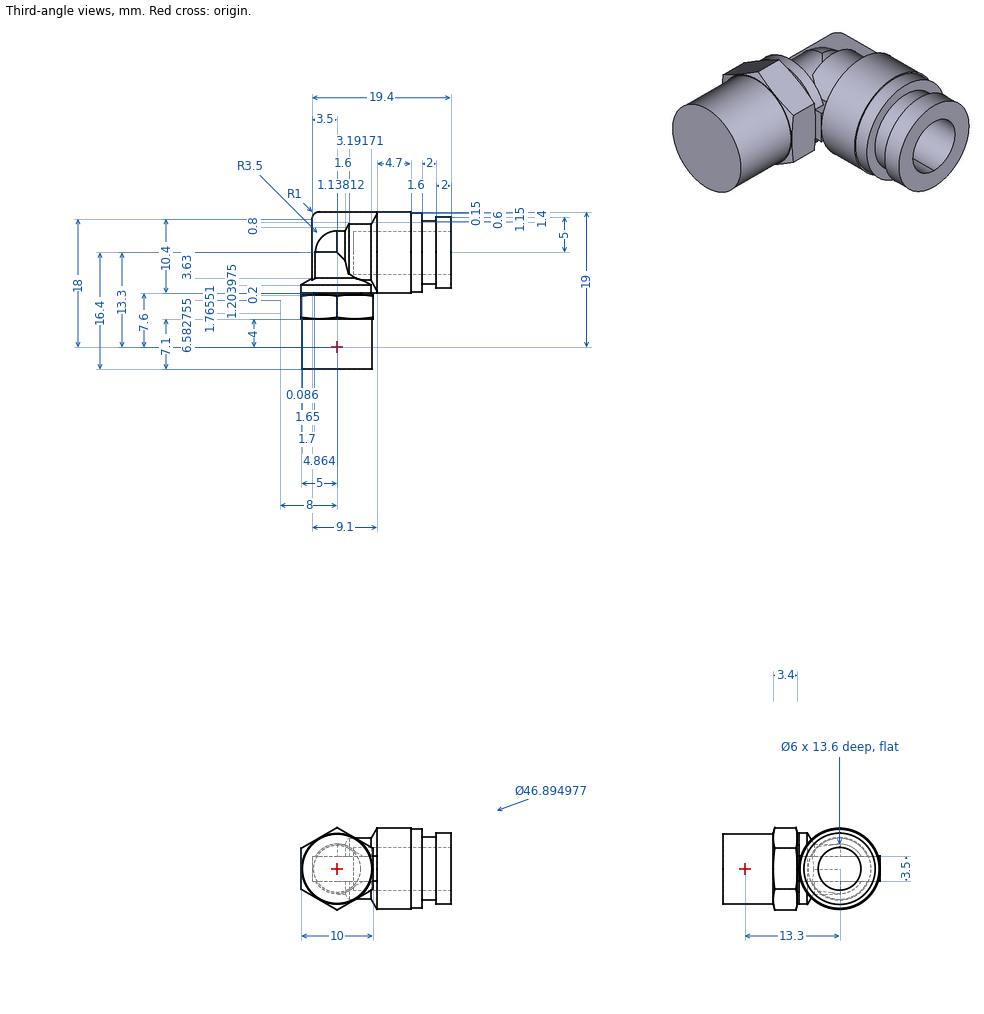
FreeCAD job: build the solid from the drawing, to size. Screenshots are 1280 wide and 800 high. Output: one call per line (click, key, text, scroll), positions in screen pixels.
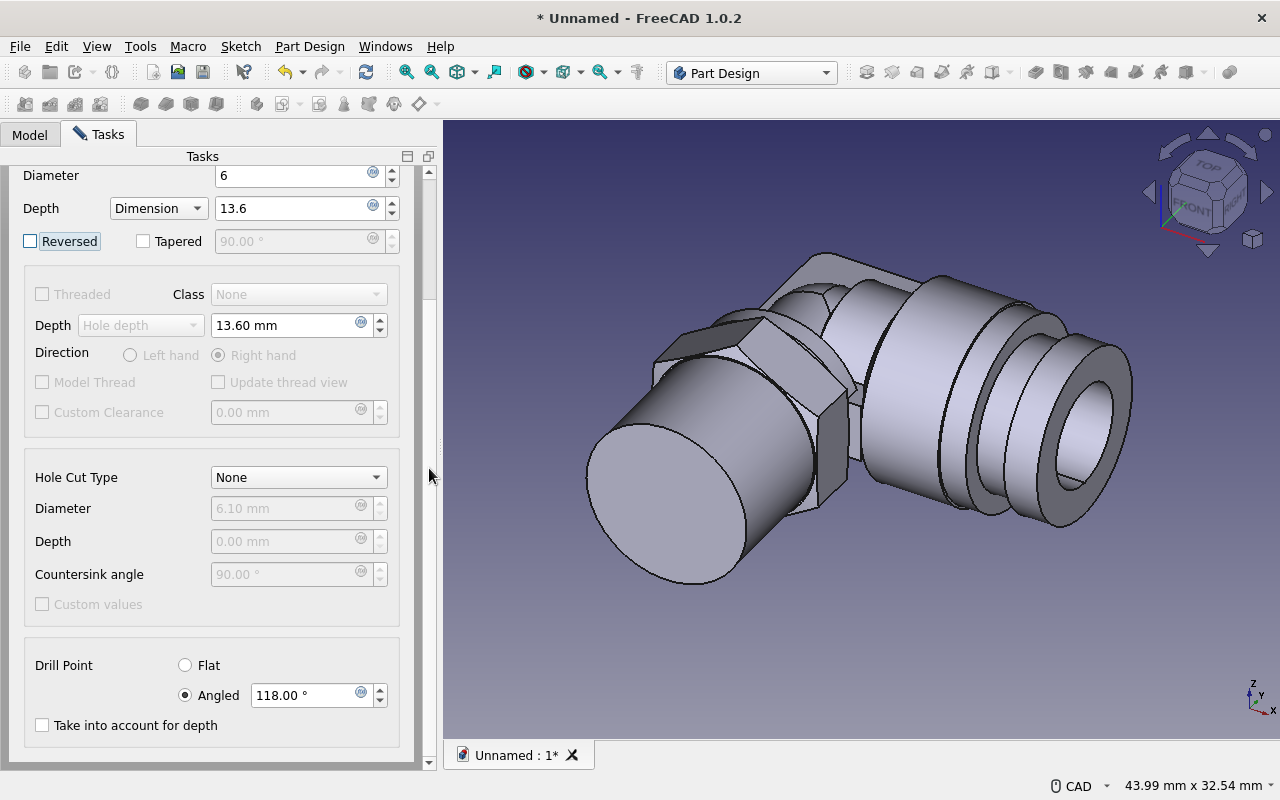
click(186, 663)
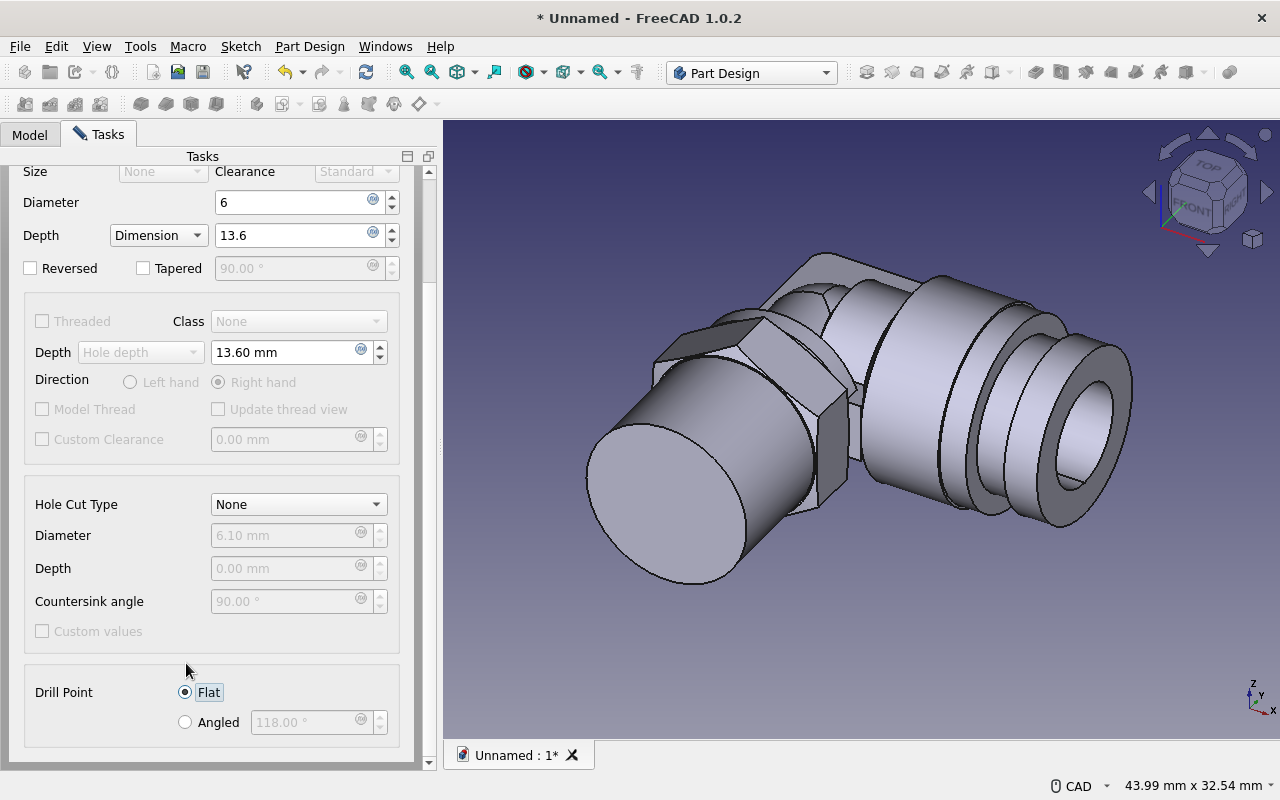
scroll(429, 468, up, 3)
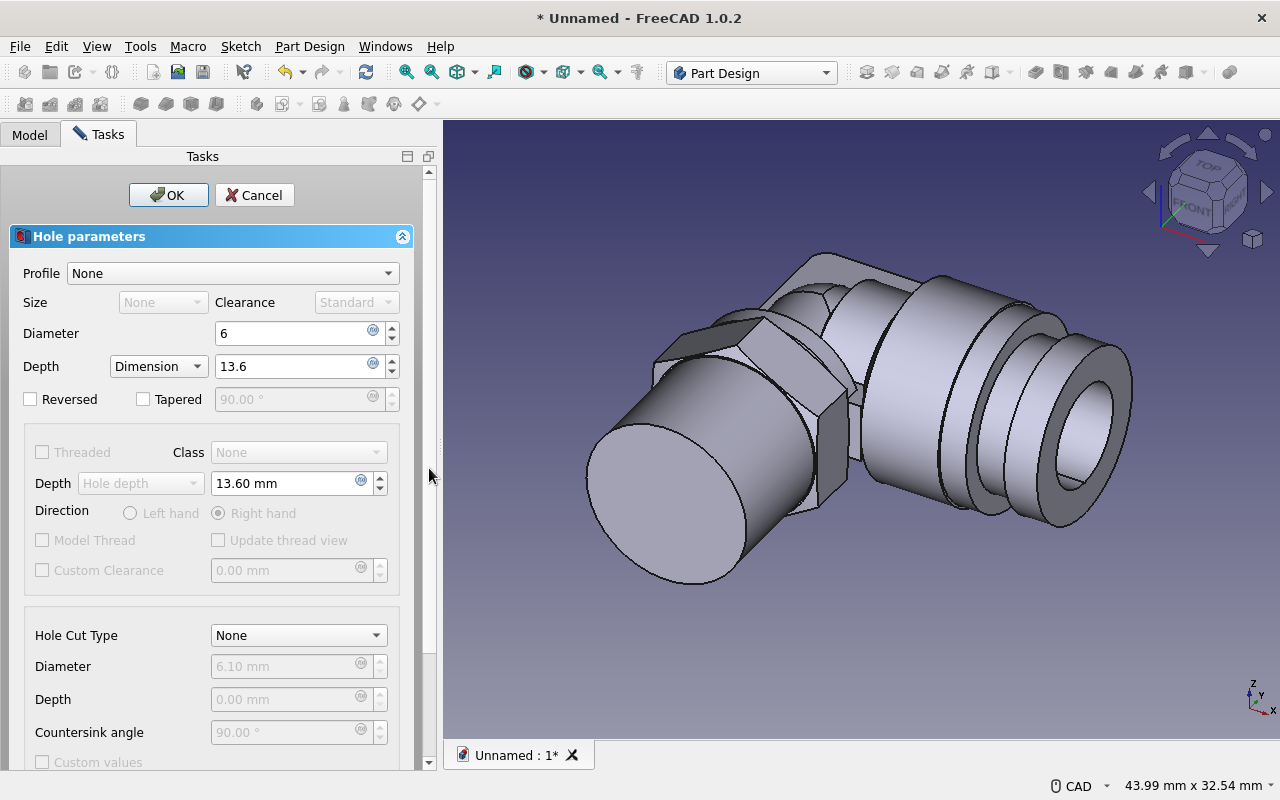
click(169, 195)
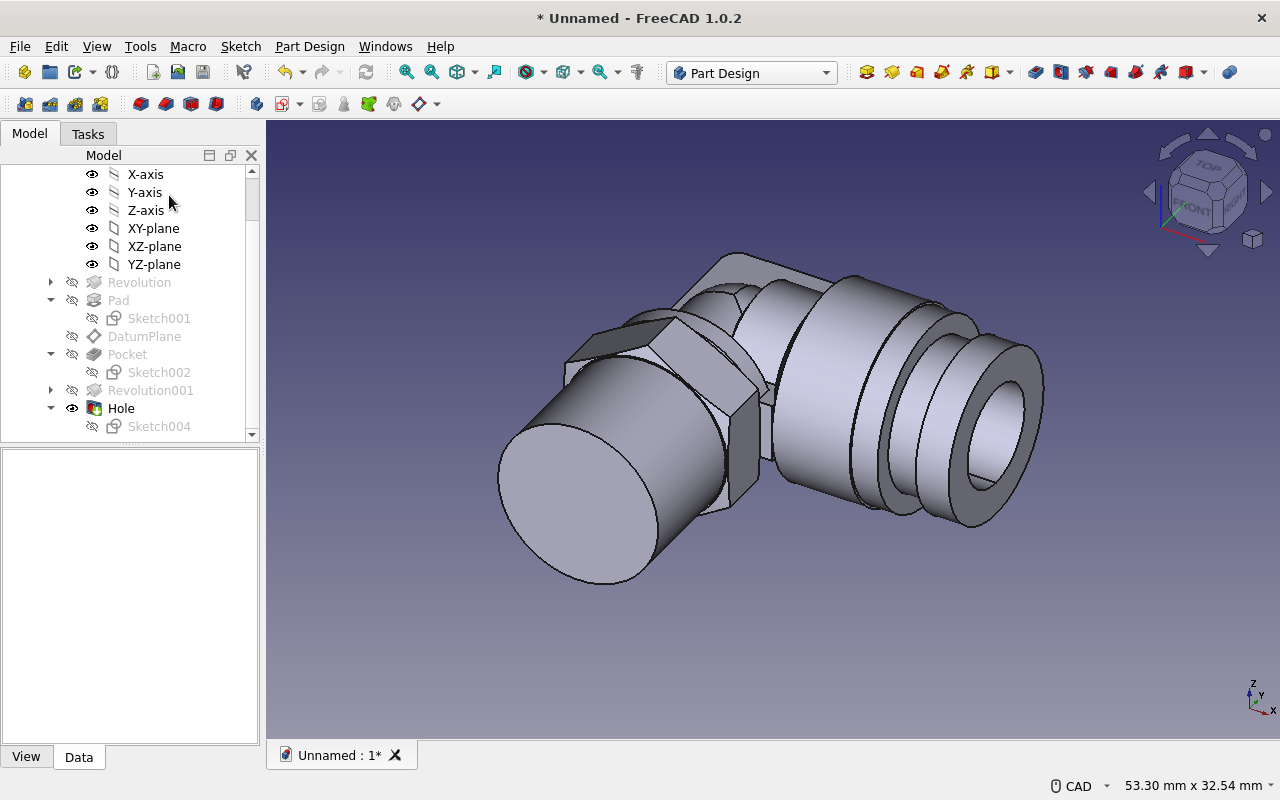
key(0)